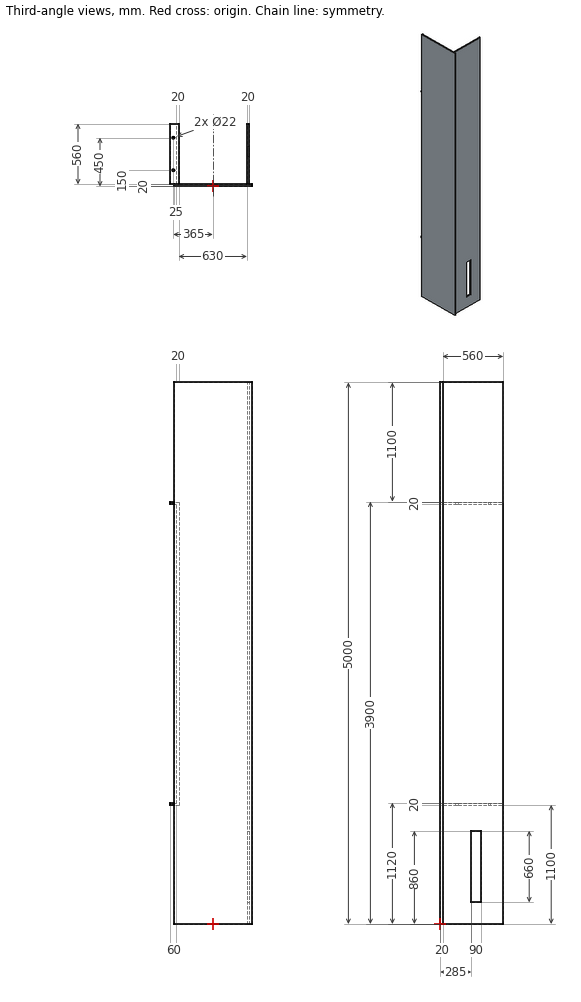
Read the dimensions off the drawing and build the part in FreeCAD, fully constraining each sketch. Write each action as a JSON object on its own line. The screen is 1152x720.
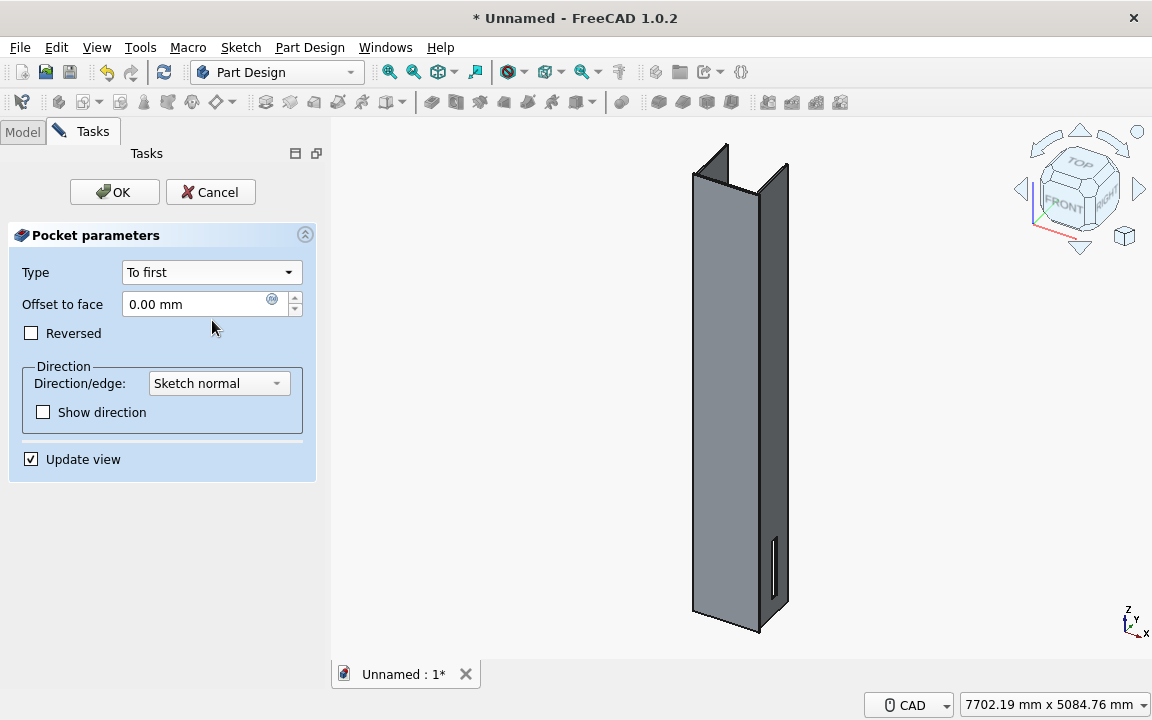
{"action": "left_click", "coordinate": [115, 192]}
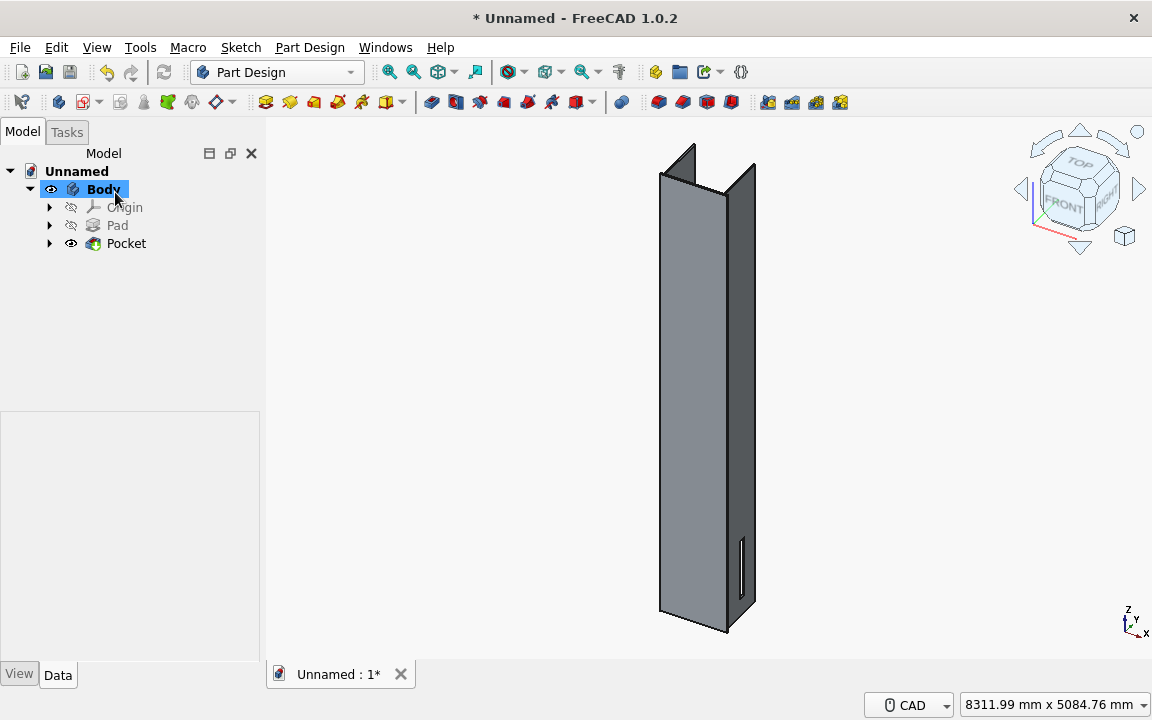
{"action": "key", "text": "6"}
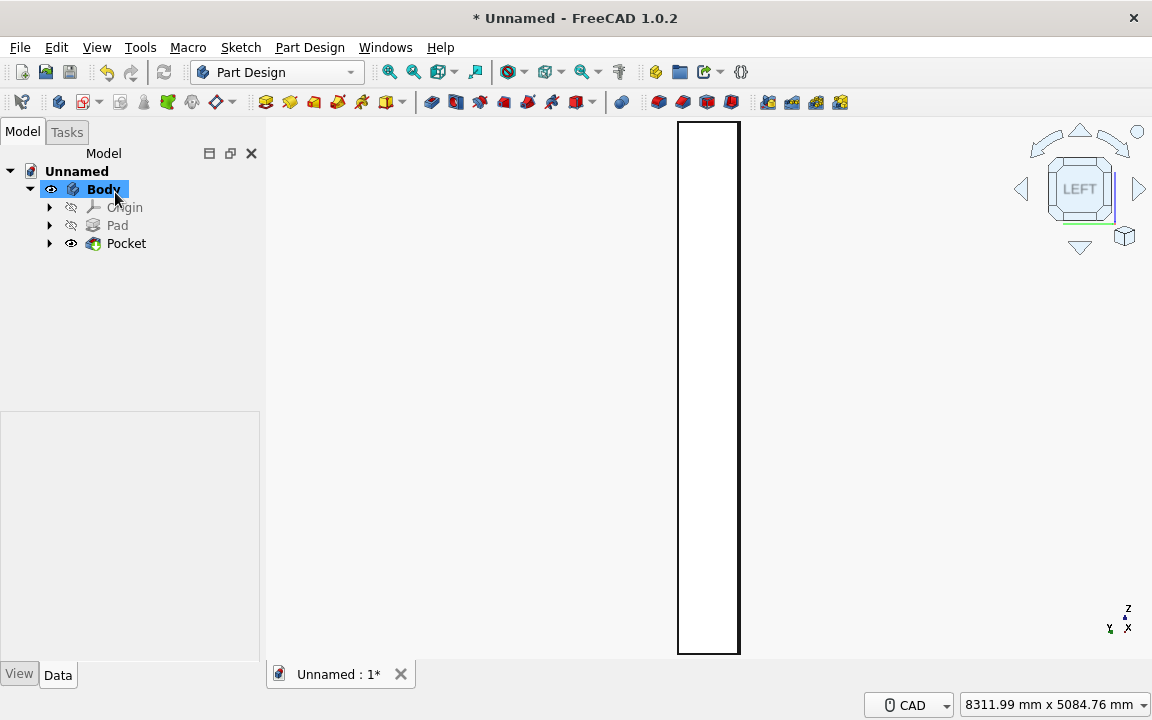
{"action": "left_click", "coordinate": [708, 159]}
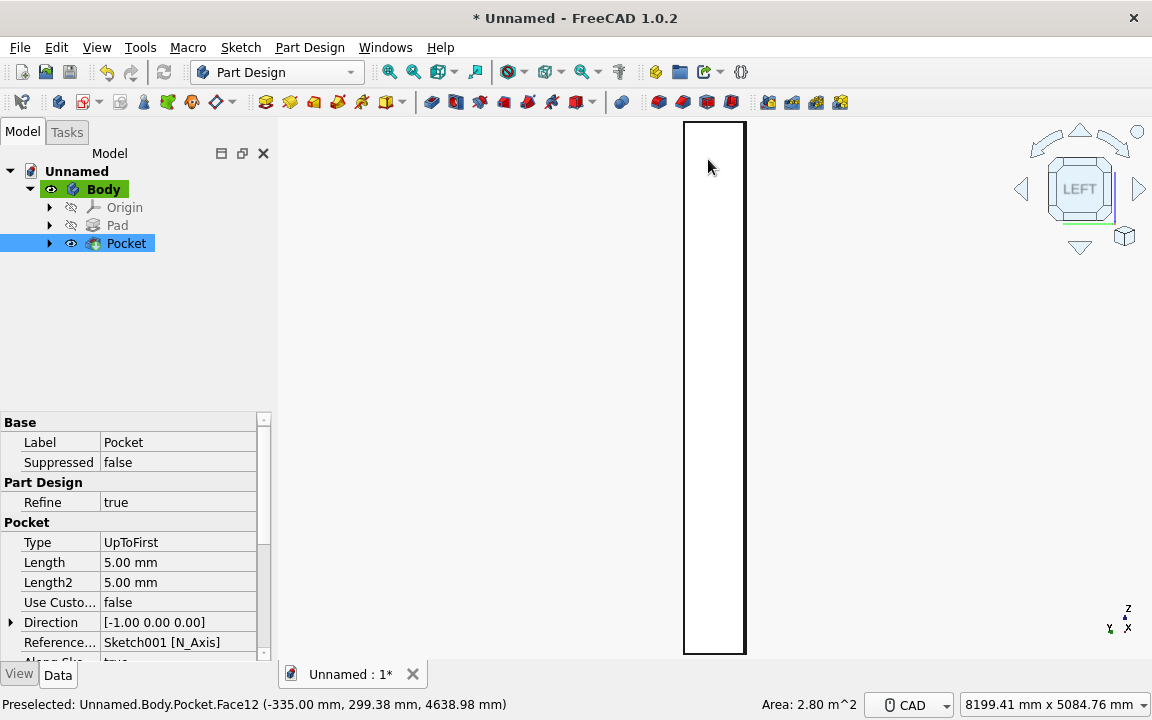
{"action": "left_click", "coordinate": [84, 102]}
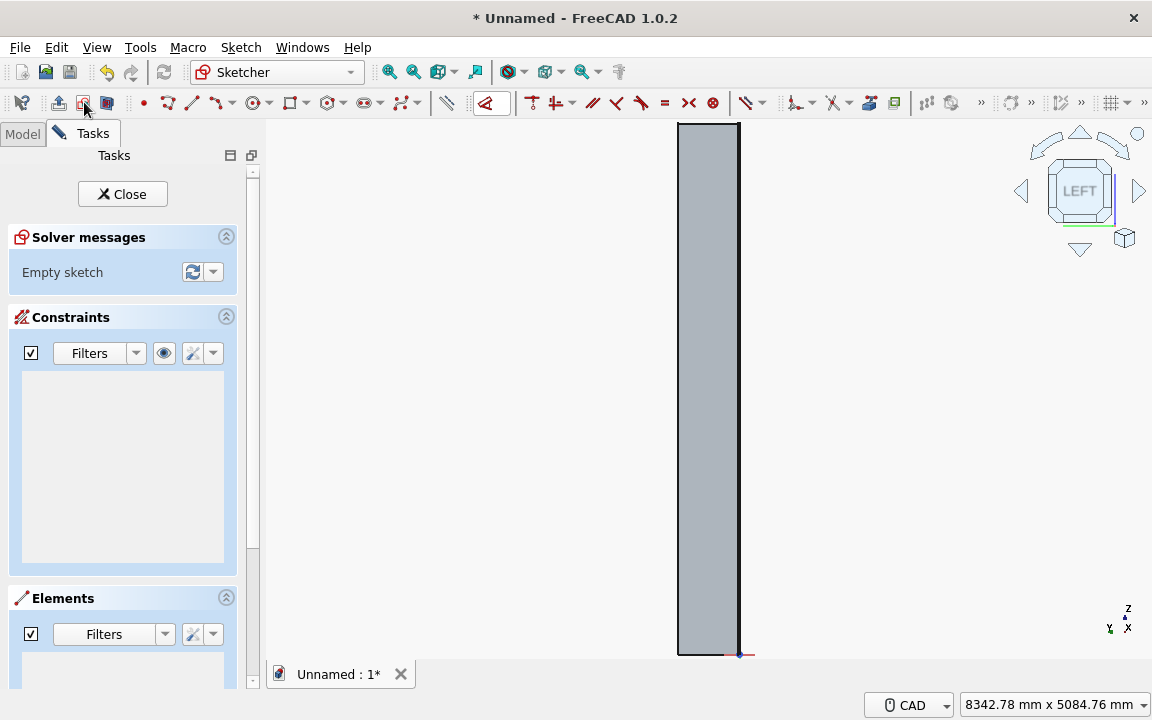
{"action": "scroll", "coordinate": [501, 389], "scroll_direction": "down", "scroll_amount": 2}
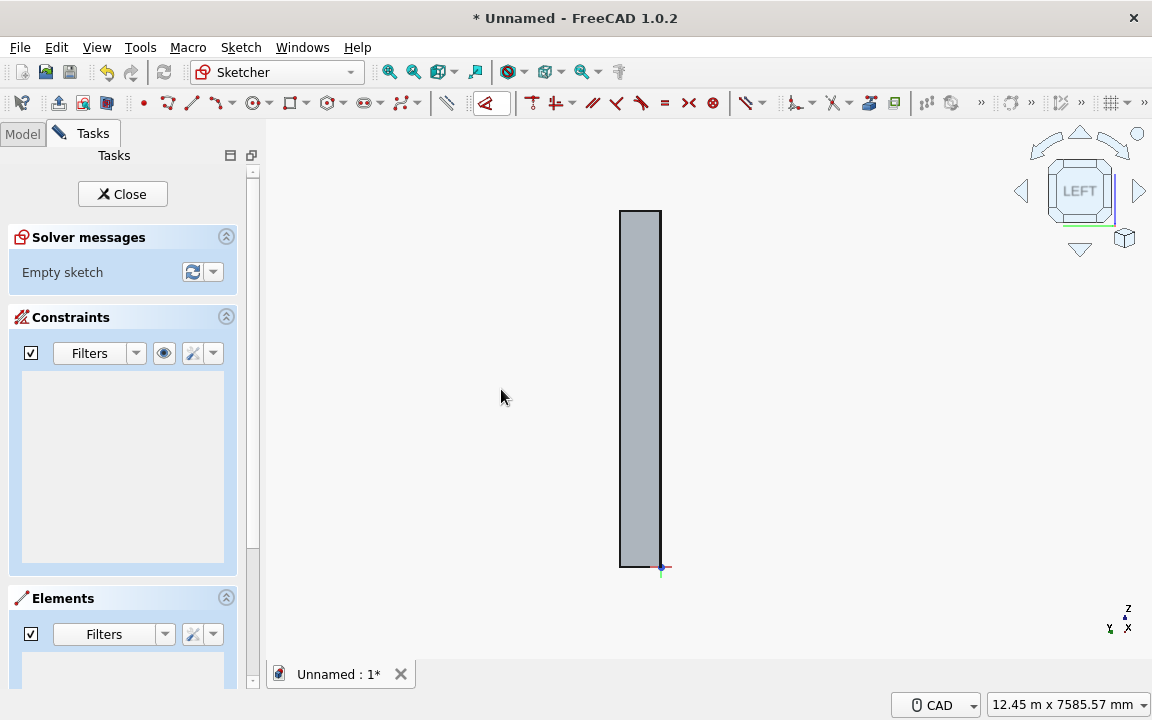
{"action": "left_click", "coordinate": [290, 104]}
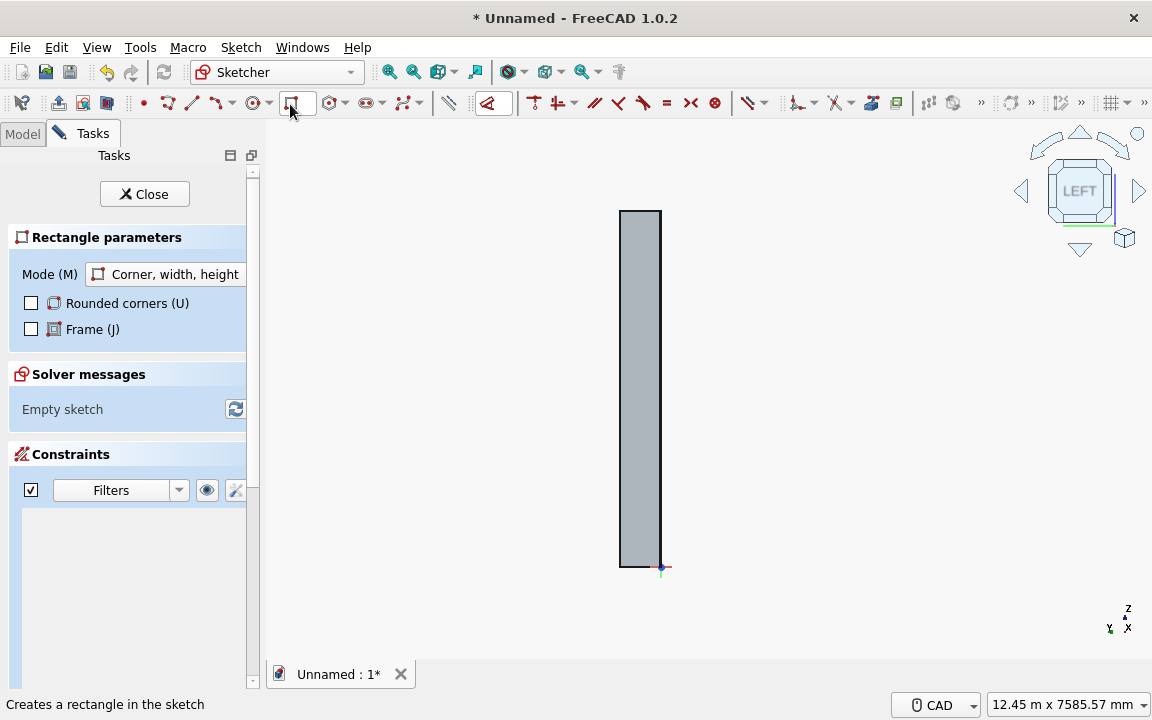
{"action": "left_click", "coordinate": [620, 211]}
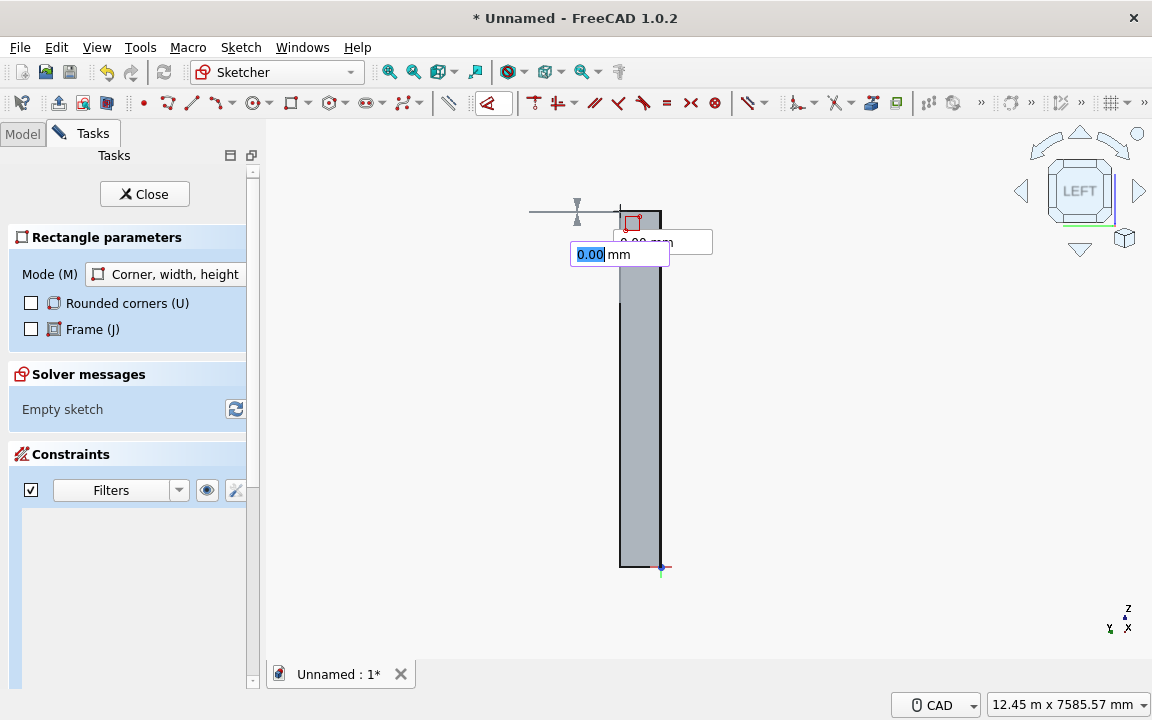
{"action": "scroll", "coordinate": [660, 290], "scroll_direction": "up", "scroll_amount": 13}
{"action": "mouse_move", "coordinate": [651, 279]}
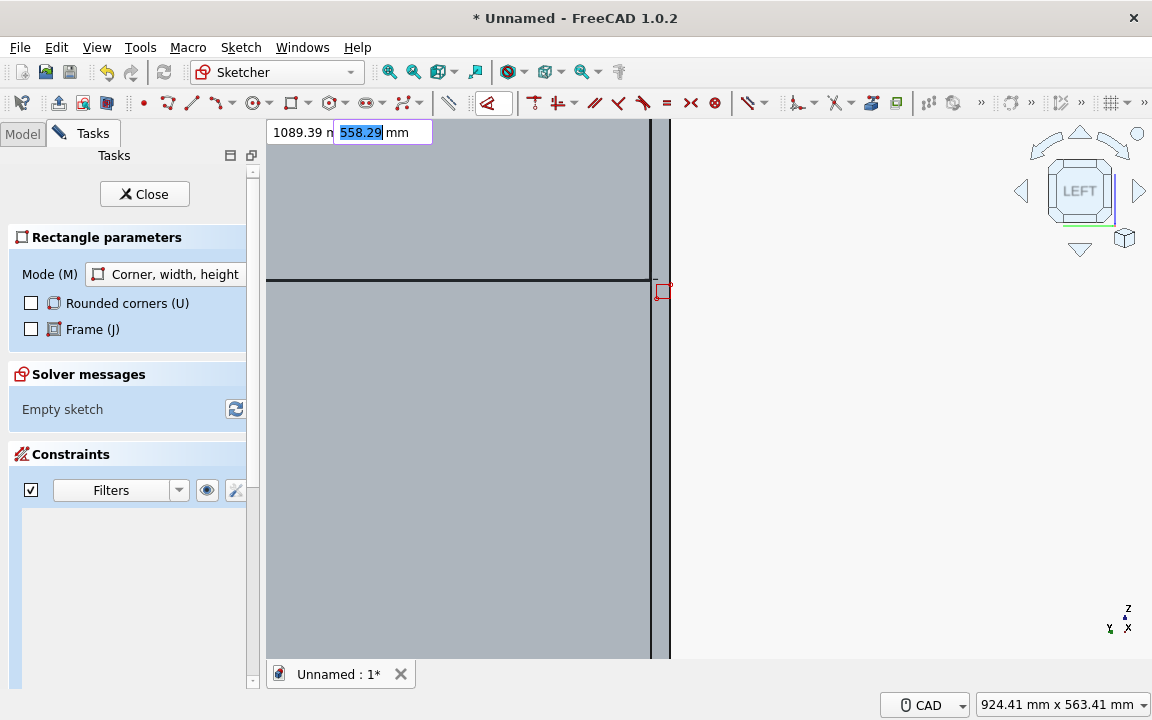
{"action": "type", "text": "560"}
{"action": "key", "text": "Tab"}
{"action": "type", "text": "1100"}
{"action": "key", "text": "Return"}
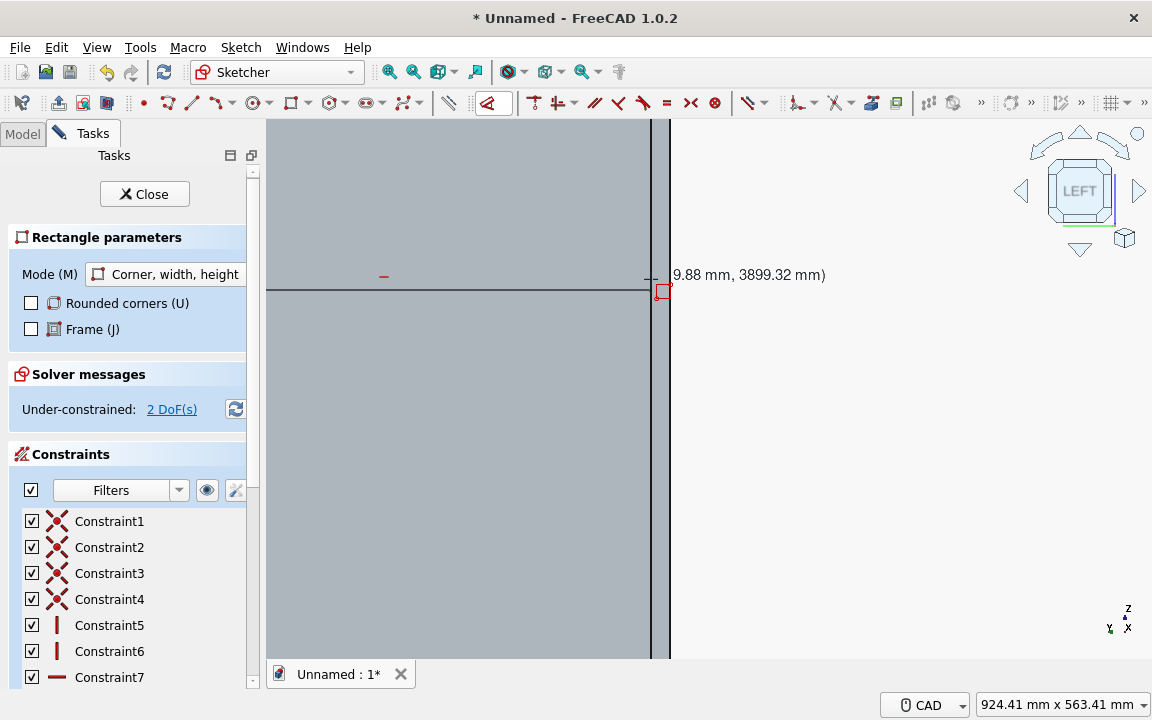
{"action": "scroll", "coordinate": [660, 290], "scroll_direction": "down", "scroll_amount": 13}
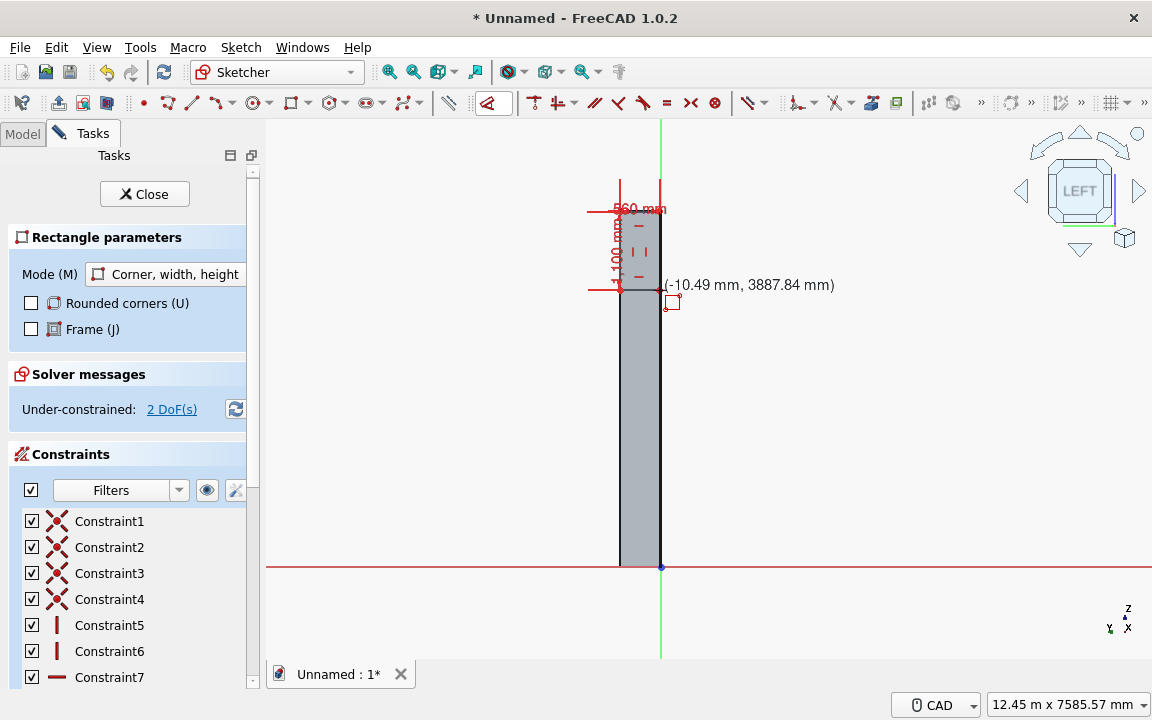
{"action": "left_click", "coordinate": [620, 489]}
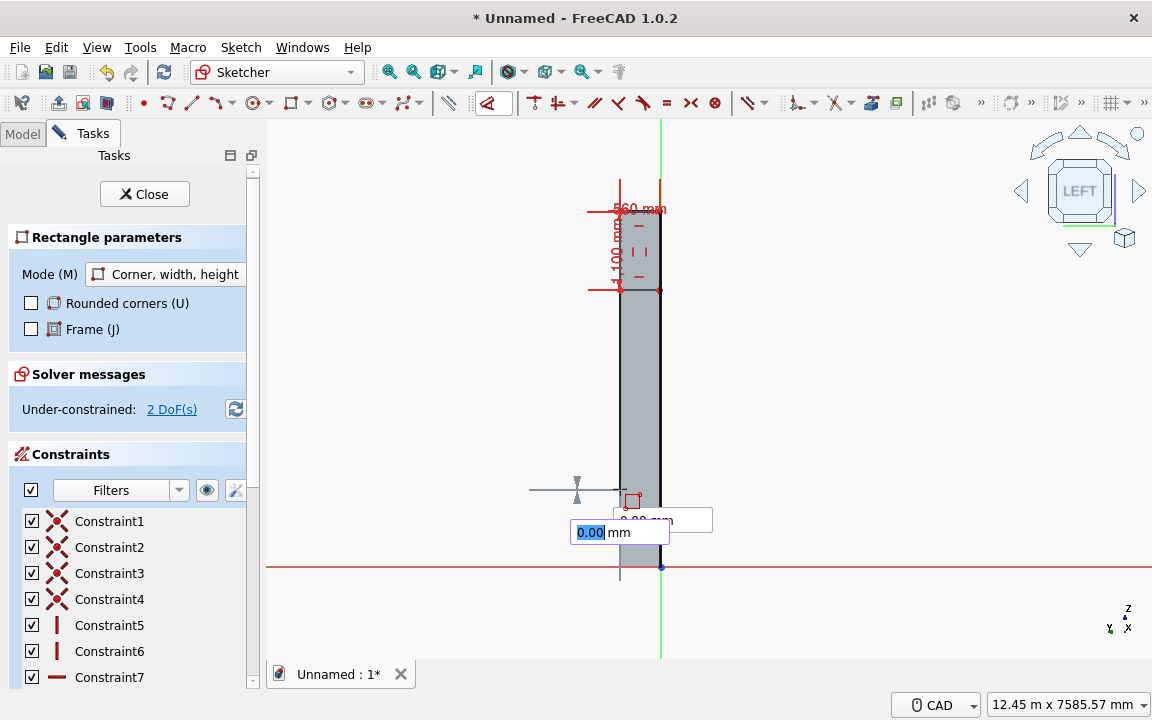
{"action": "scroll", "coordinate": [660, 567], "scroll_direction": "up", "scroll_amount": 13}